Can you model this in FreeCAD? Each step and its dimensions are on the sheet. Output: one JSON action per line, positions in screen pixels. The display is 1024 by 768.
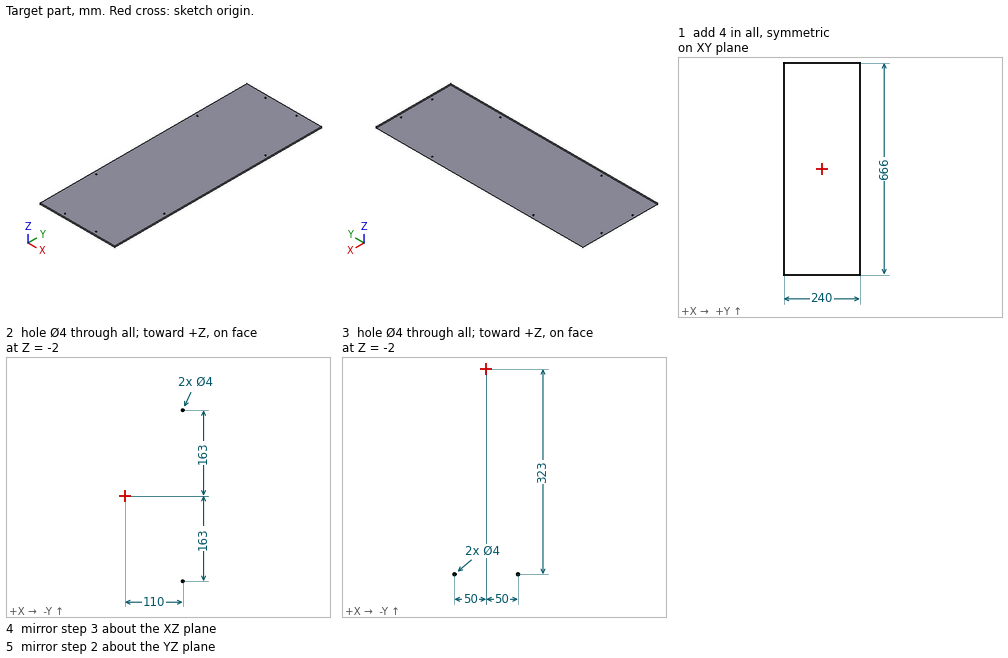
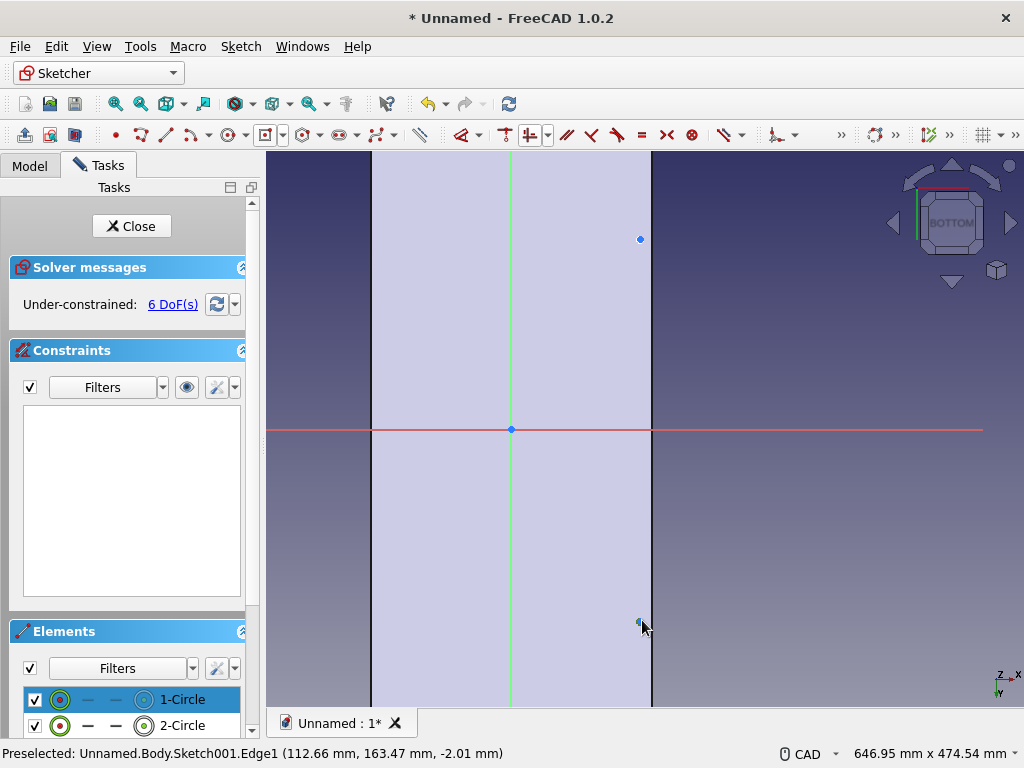
{"action": "scroll", "coordinate": [642, 238], "scroll_direction": "up", "scroll_amount": 8}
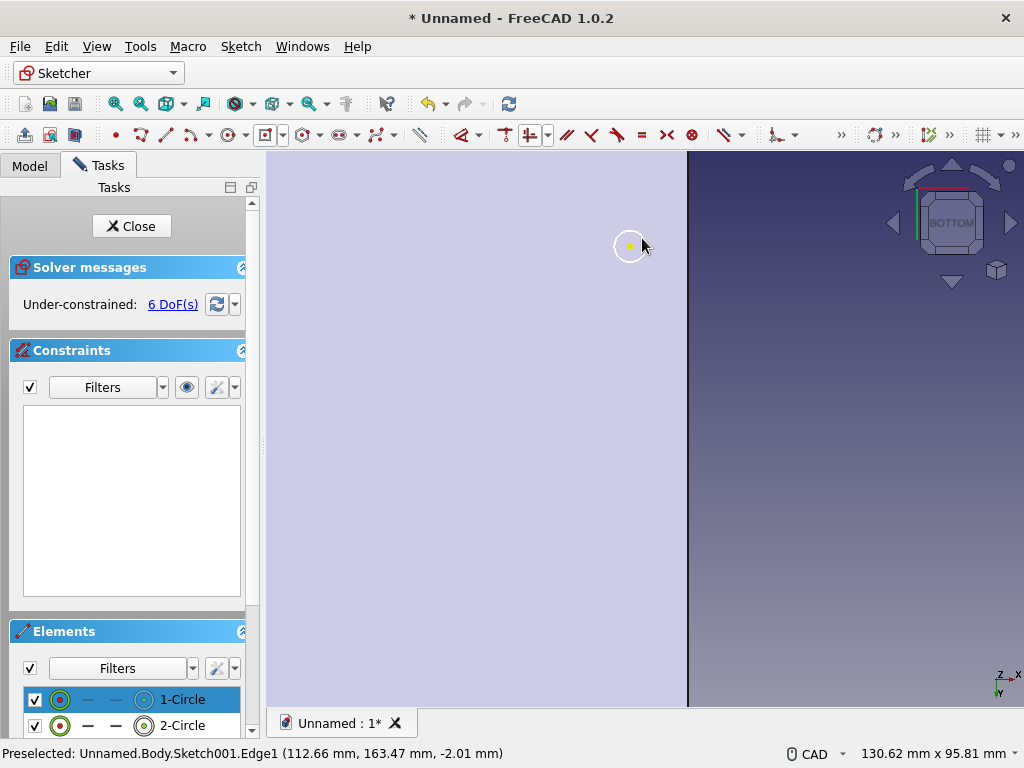
{"action": "left_click", "coordinate": [641, 235]}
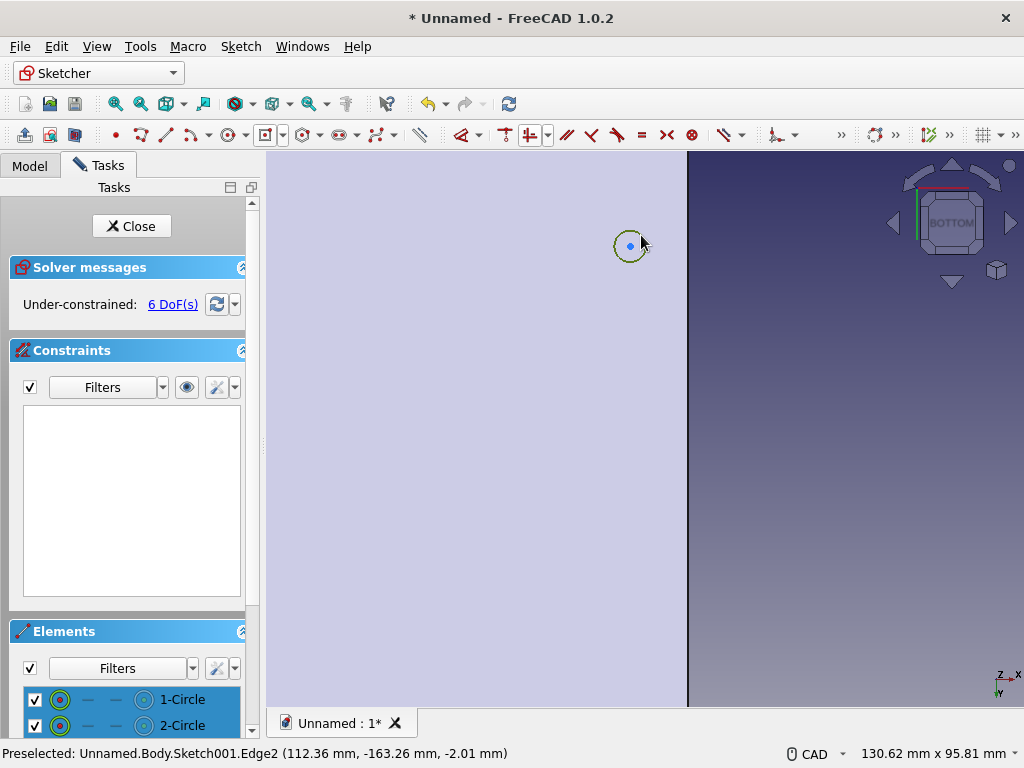
{"action": "left_click", "coordinate": [642, 136]}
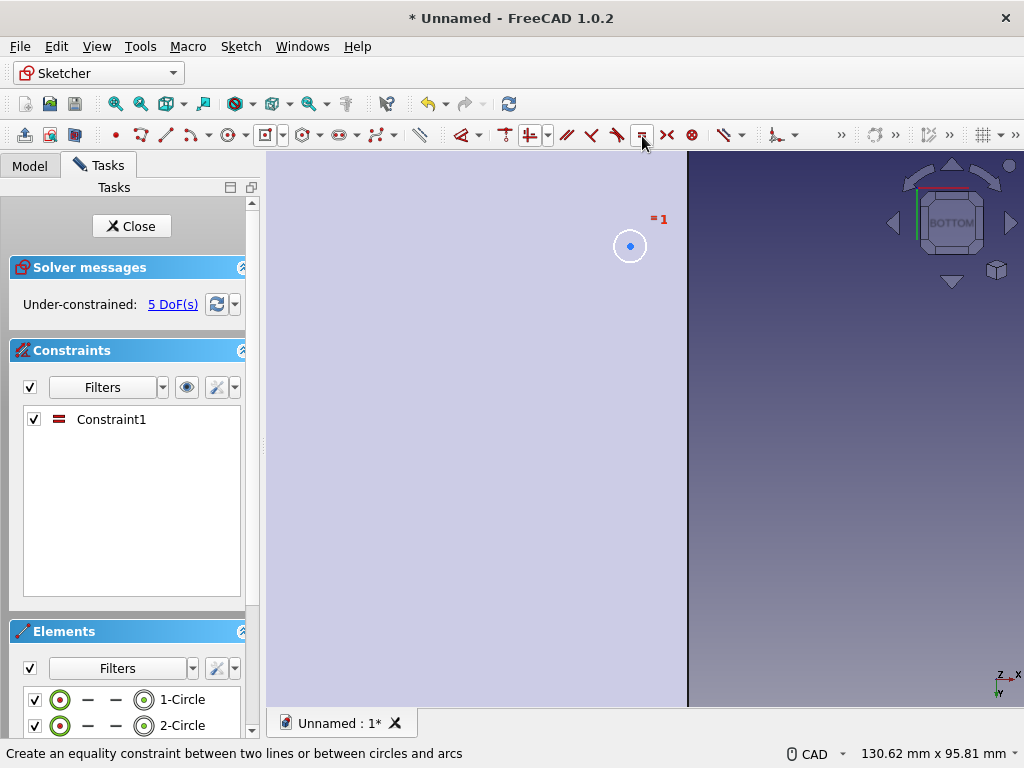
{"action": "scroll", "coordinate": [642, 237], "scroll_direction": "down", "scroll_amount": 8}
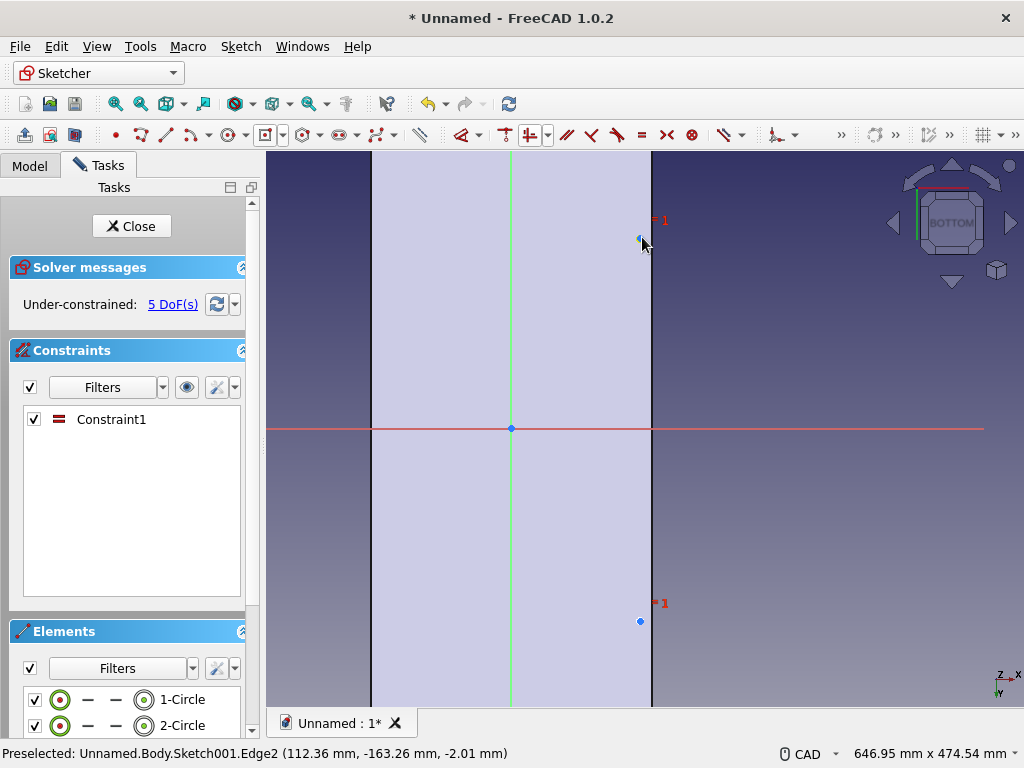
{"action": "left_click", "coordinate": [640, 621]}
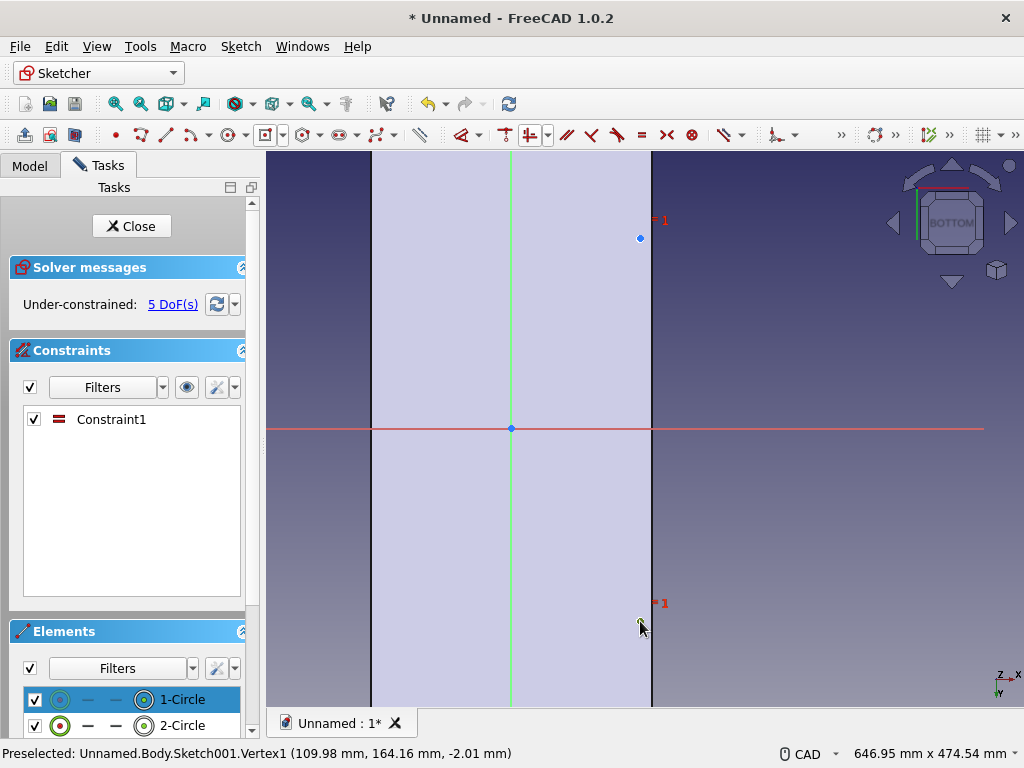
{"action": "left_click", "coordinate": [640, 239]}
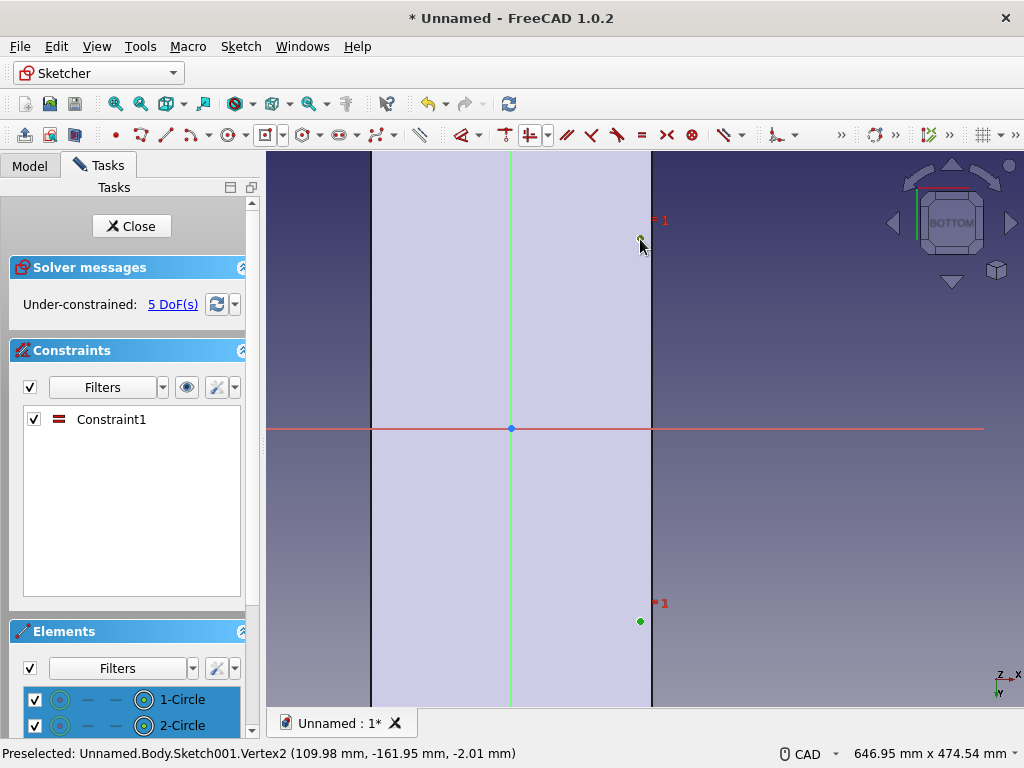
{"action": "key", "text": "v"}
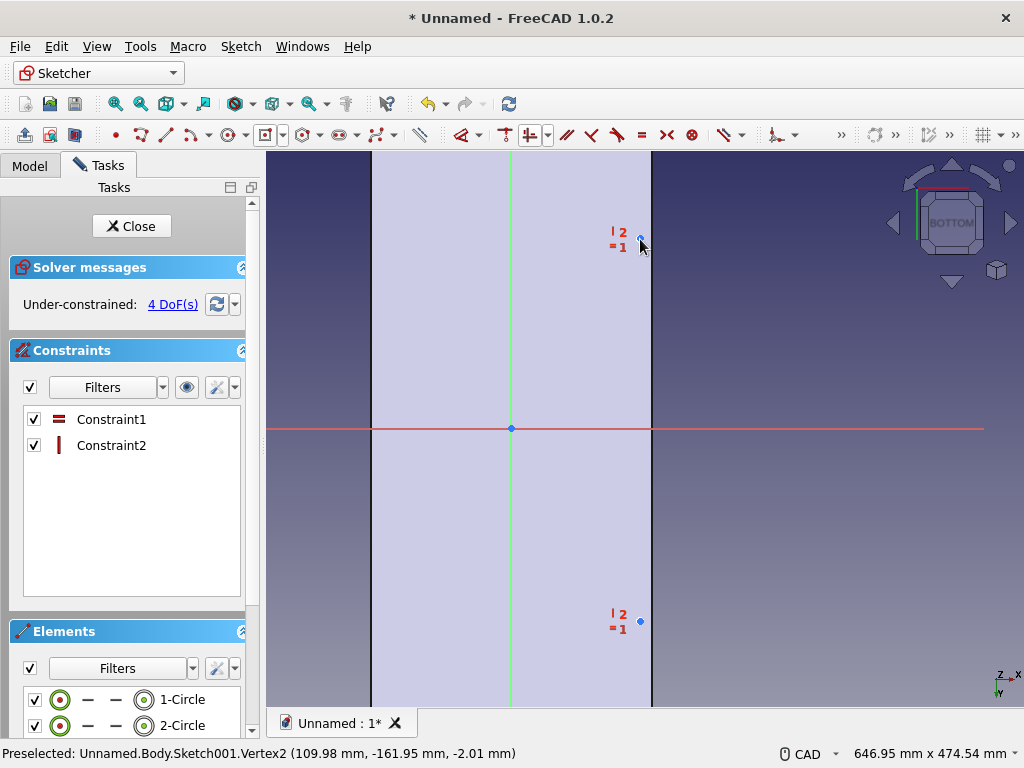
{"action": "left_click", "coordinate": [460, 136]}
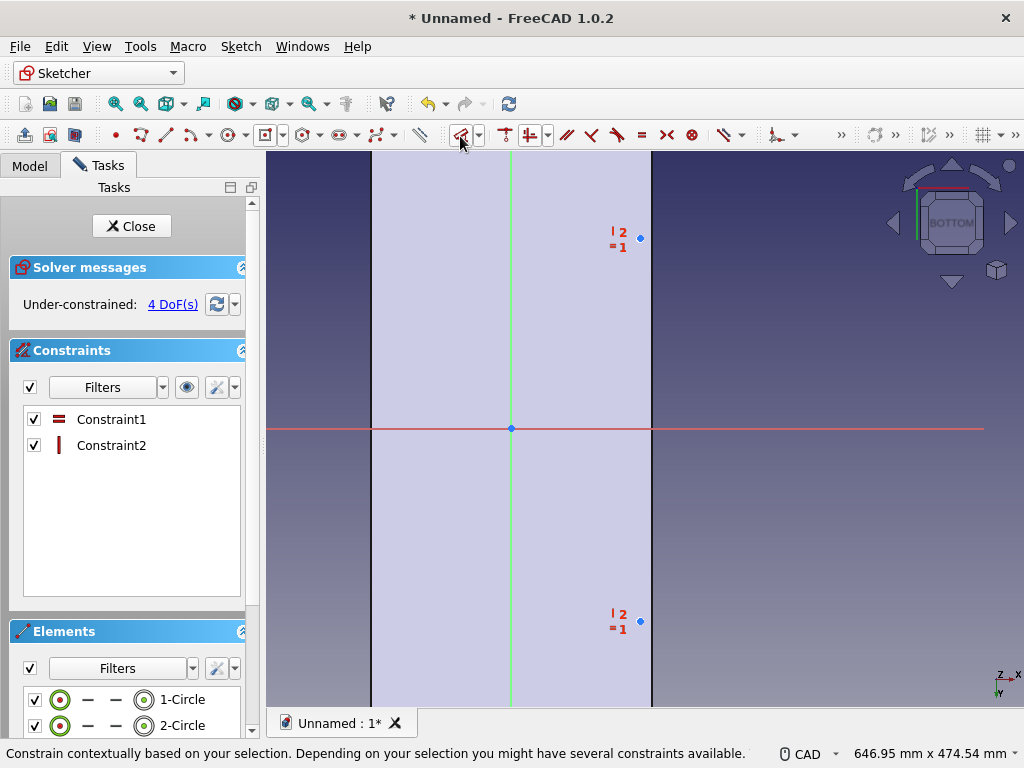
{"action": "scroll", "coordinate": [640, 618], "scroll_direction": "up", "scroll_amount": 11}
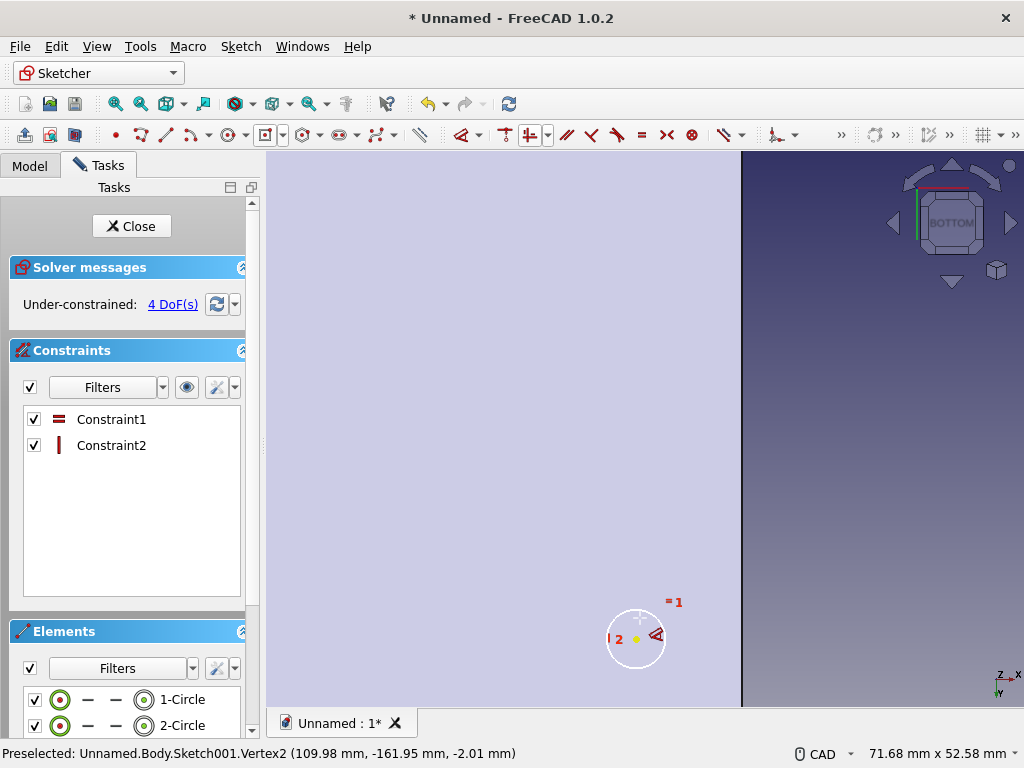
{"action": "left_click", "coordinate": [637, 610]}
{"action": "left_click", "coordinate": [638, 578]}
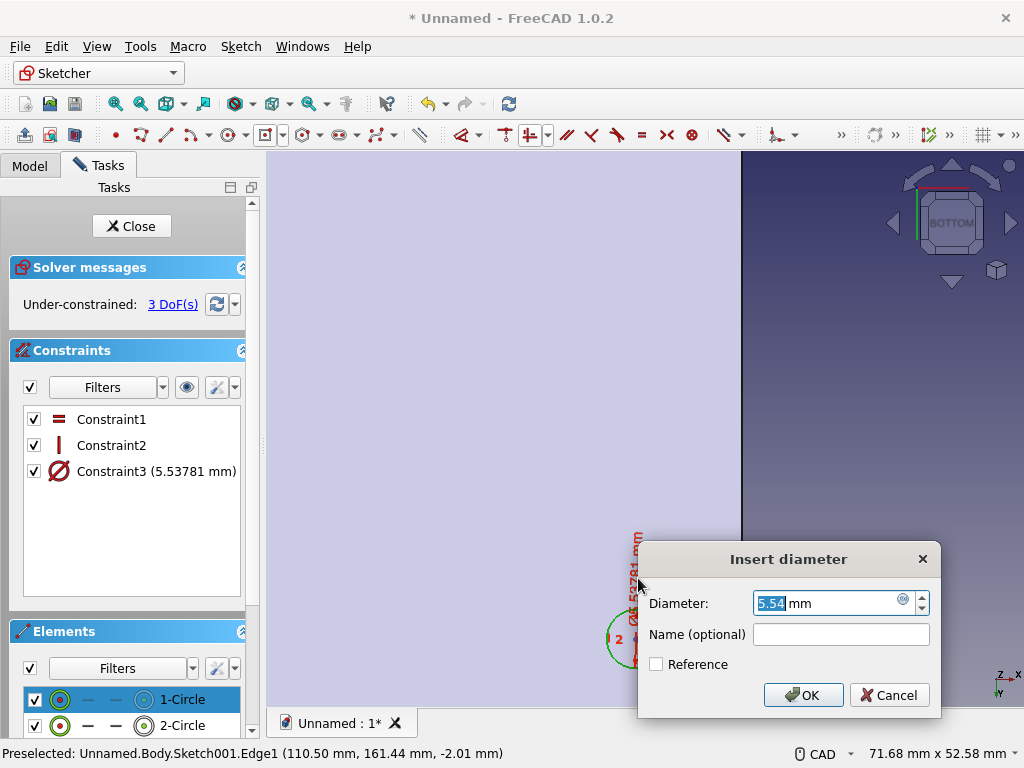
{"action": "type", "text": "4"}
{"action": "key", "text": "Return"}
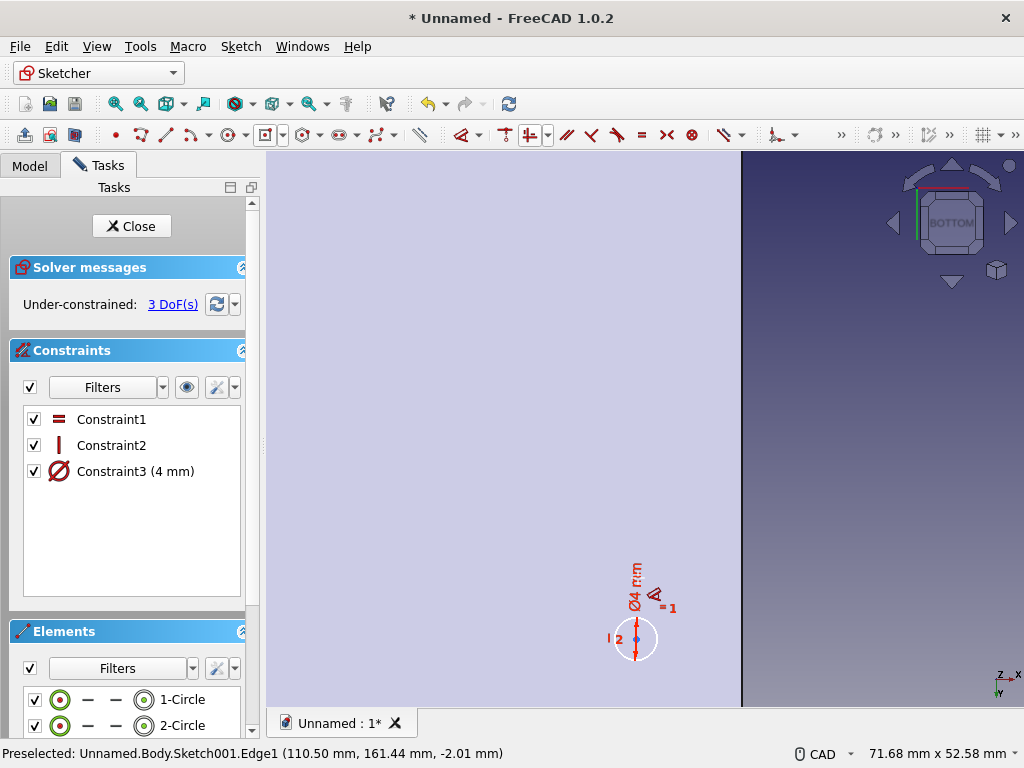
{"action": "scroll", "coordinate": [640, 619], "scroll_direction": "down", "scroll_amount": 11}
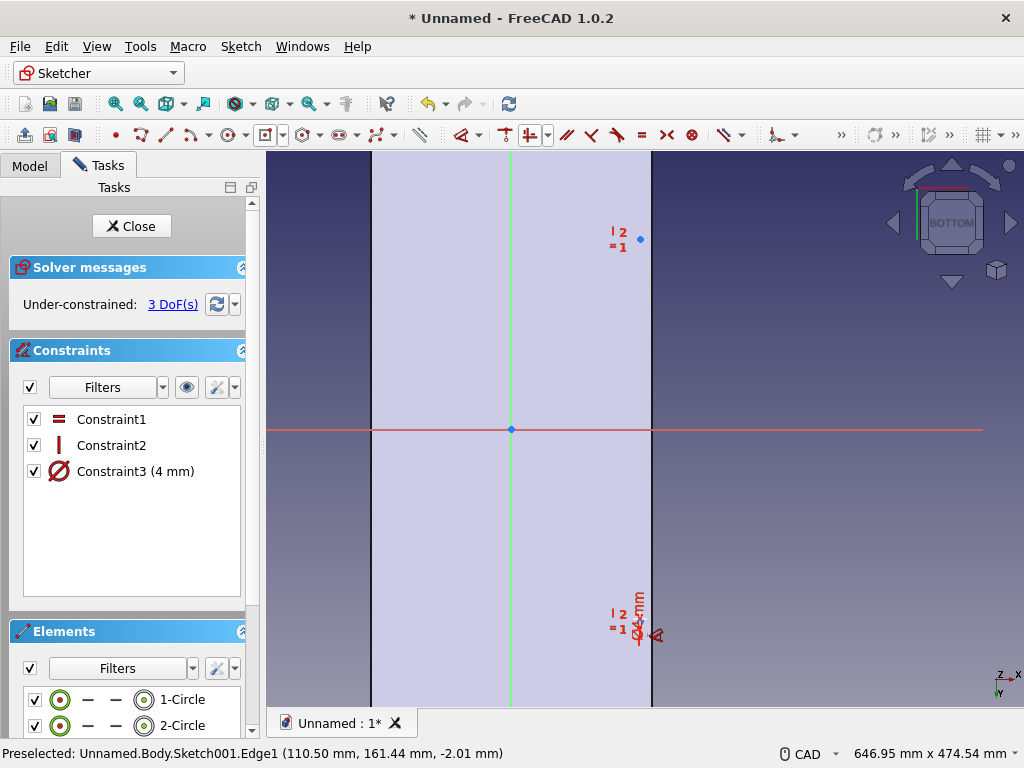
{"action": "left_click", "coordinate": [640, 622]}
{"action": "left_click", "coordinate": [576, 656]}